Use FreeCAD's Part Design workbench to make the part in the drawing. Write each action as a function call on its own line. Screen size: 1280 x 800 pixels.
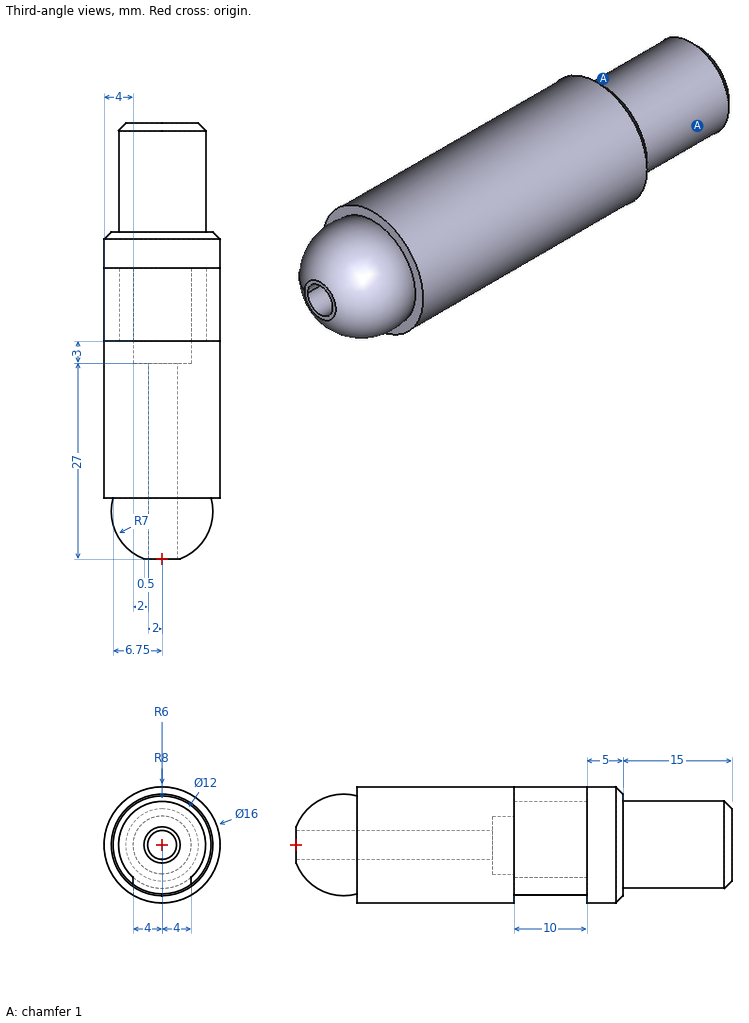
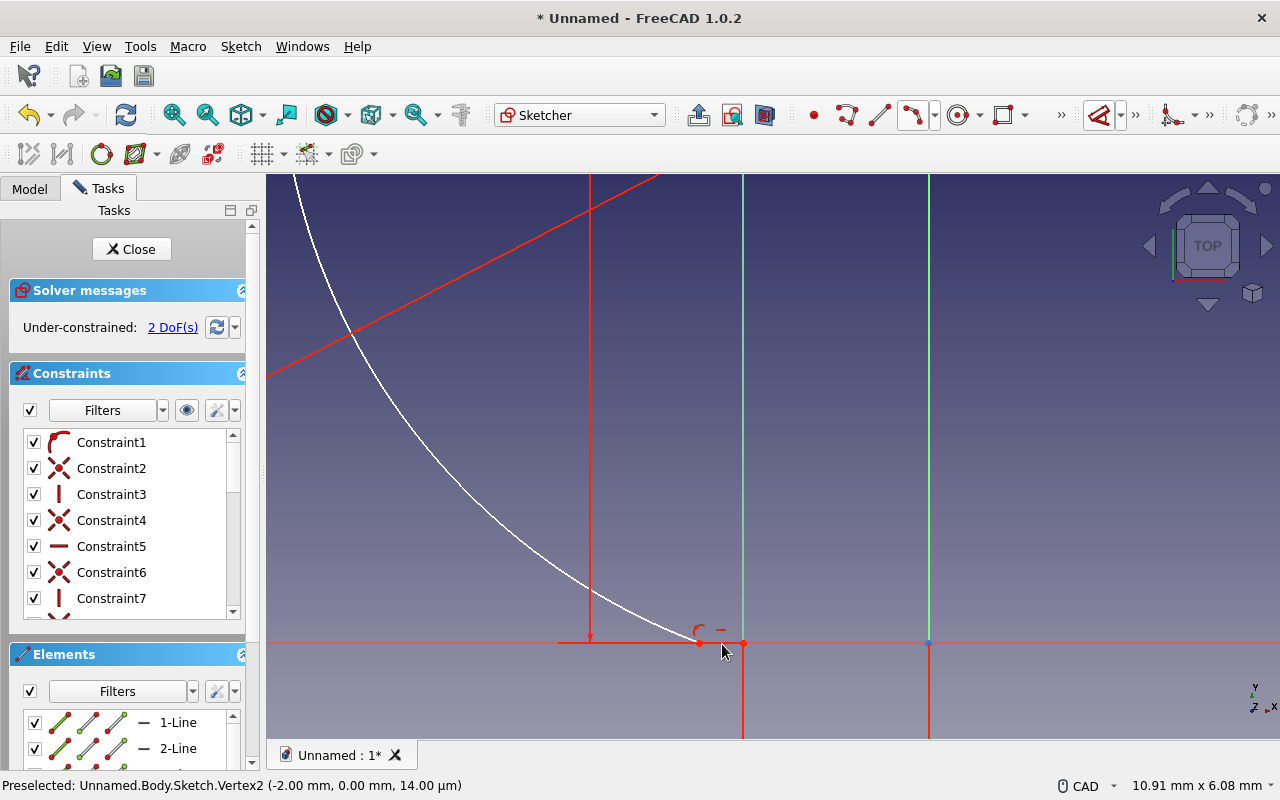
click(722, 643)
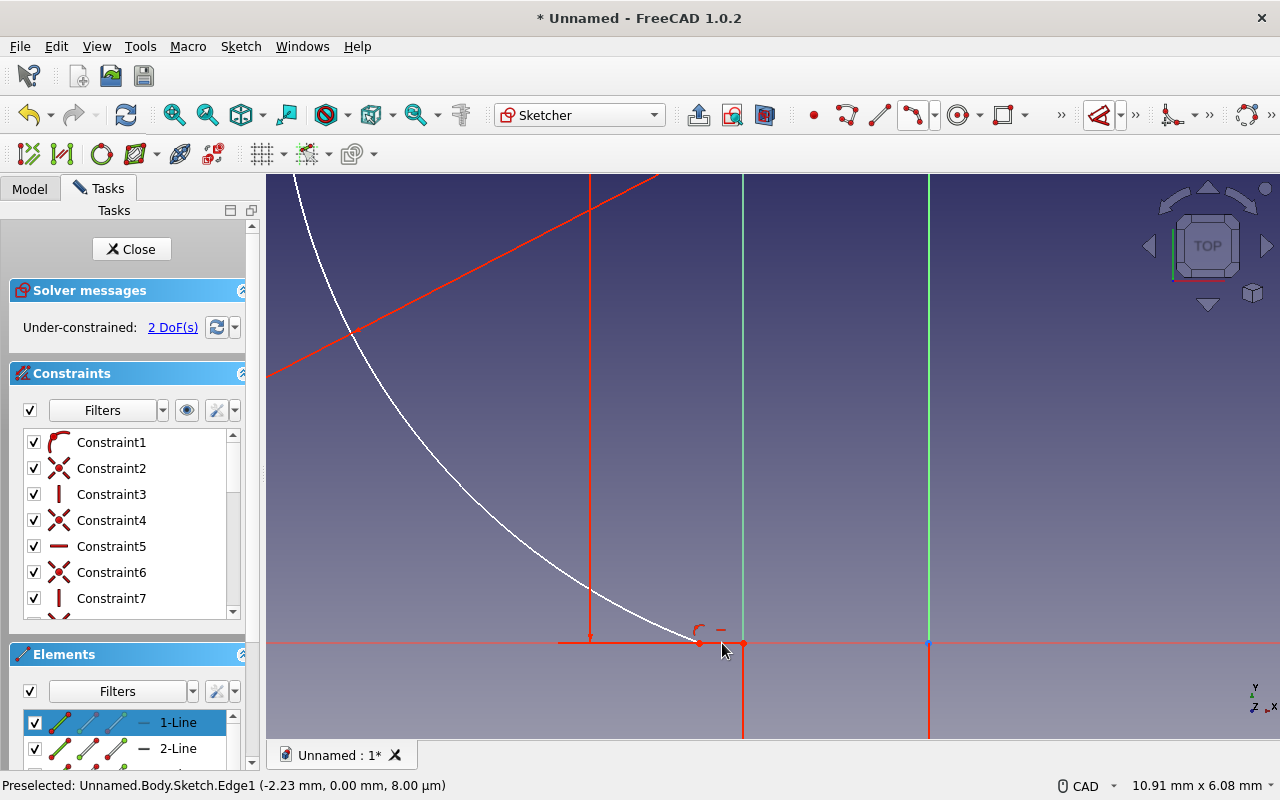
click(1120, 116)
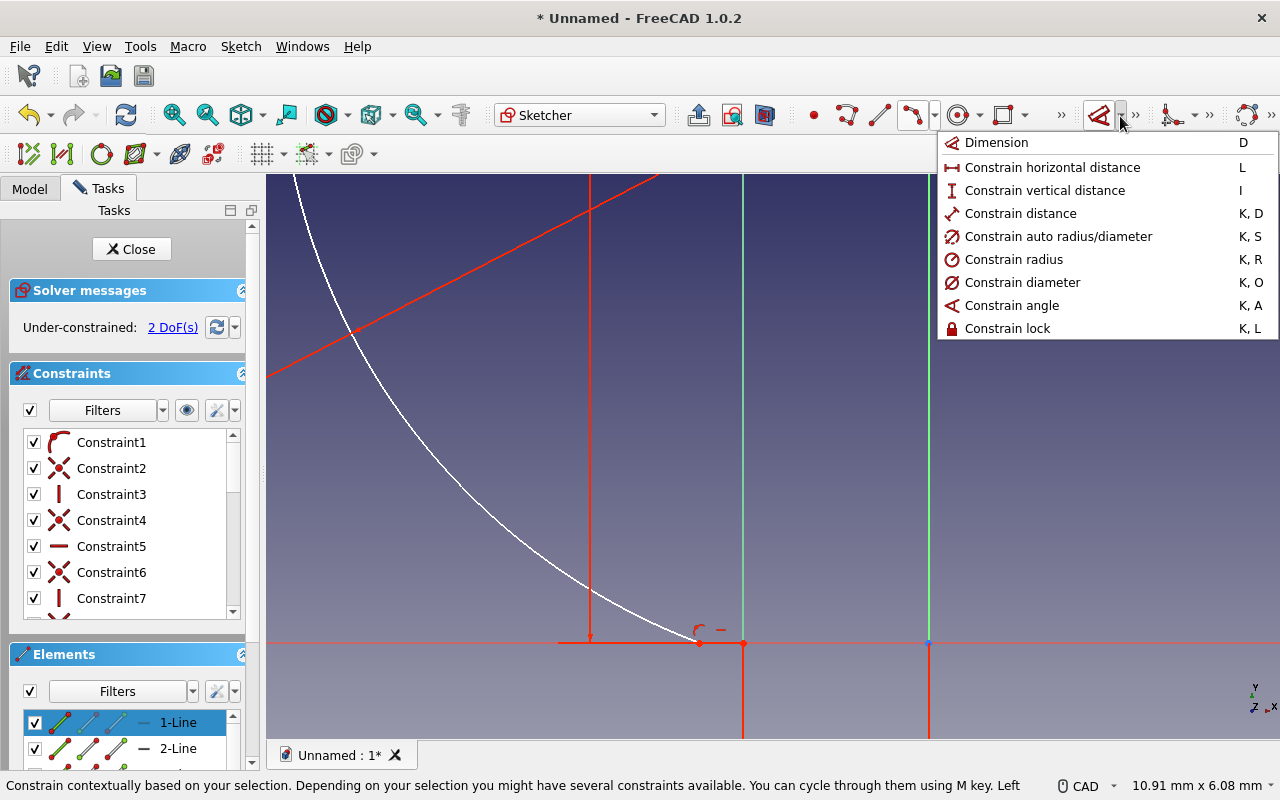
click(1108, 168)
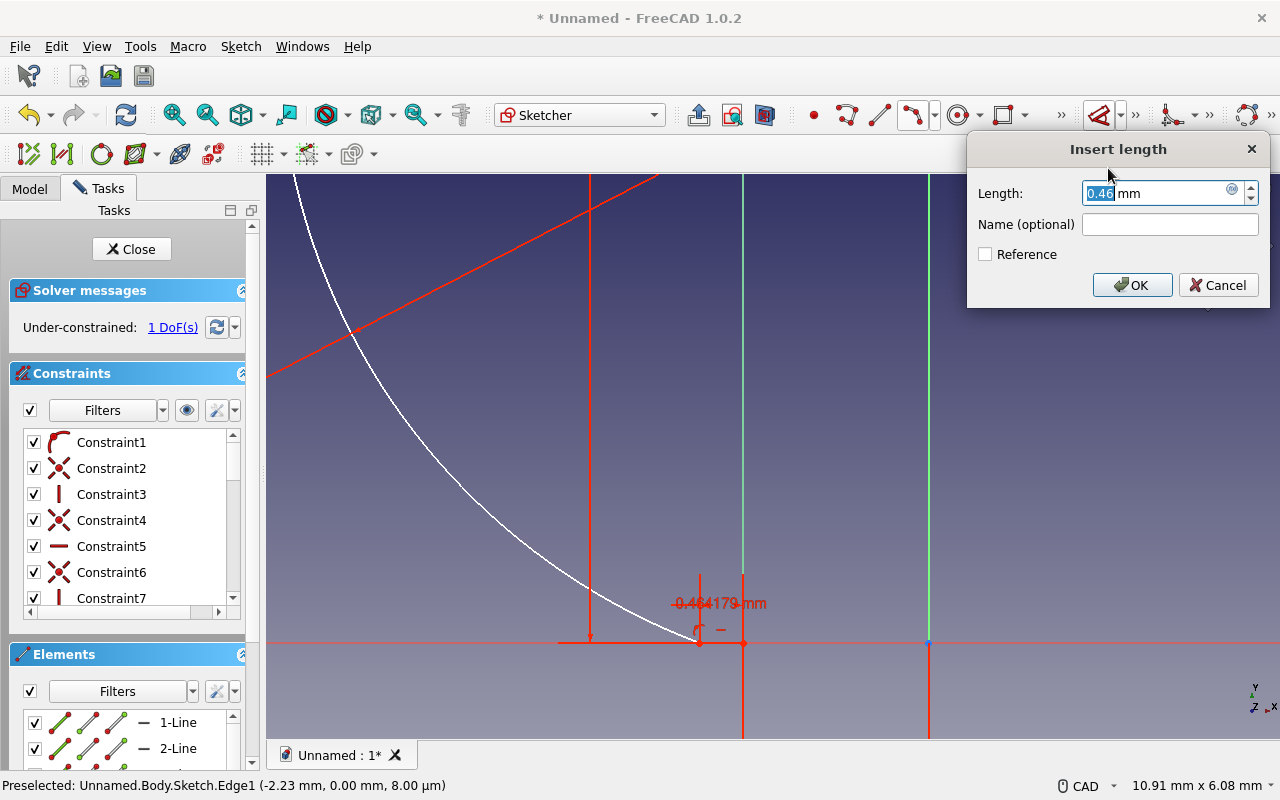
text(0.5)
key(Return)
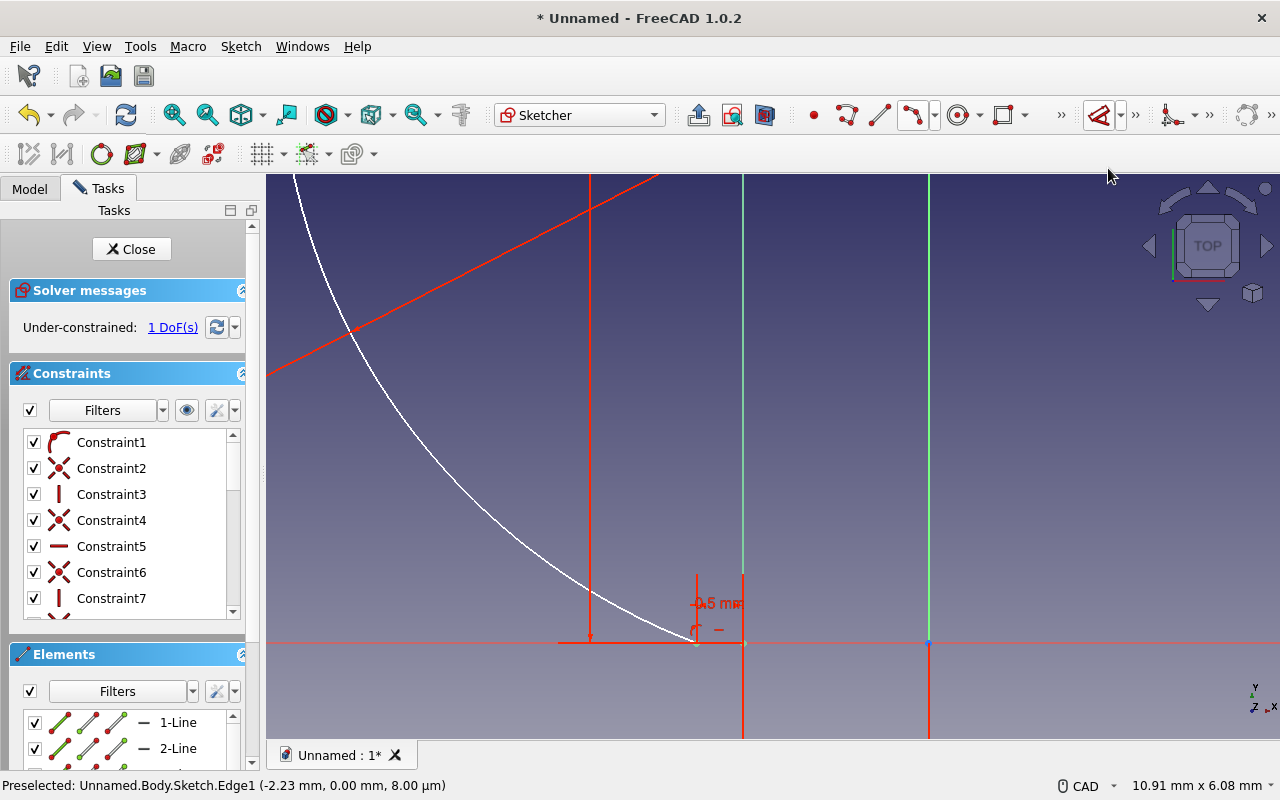
scroll(728, 645, down, 10)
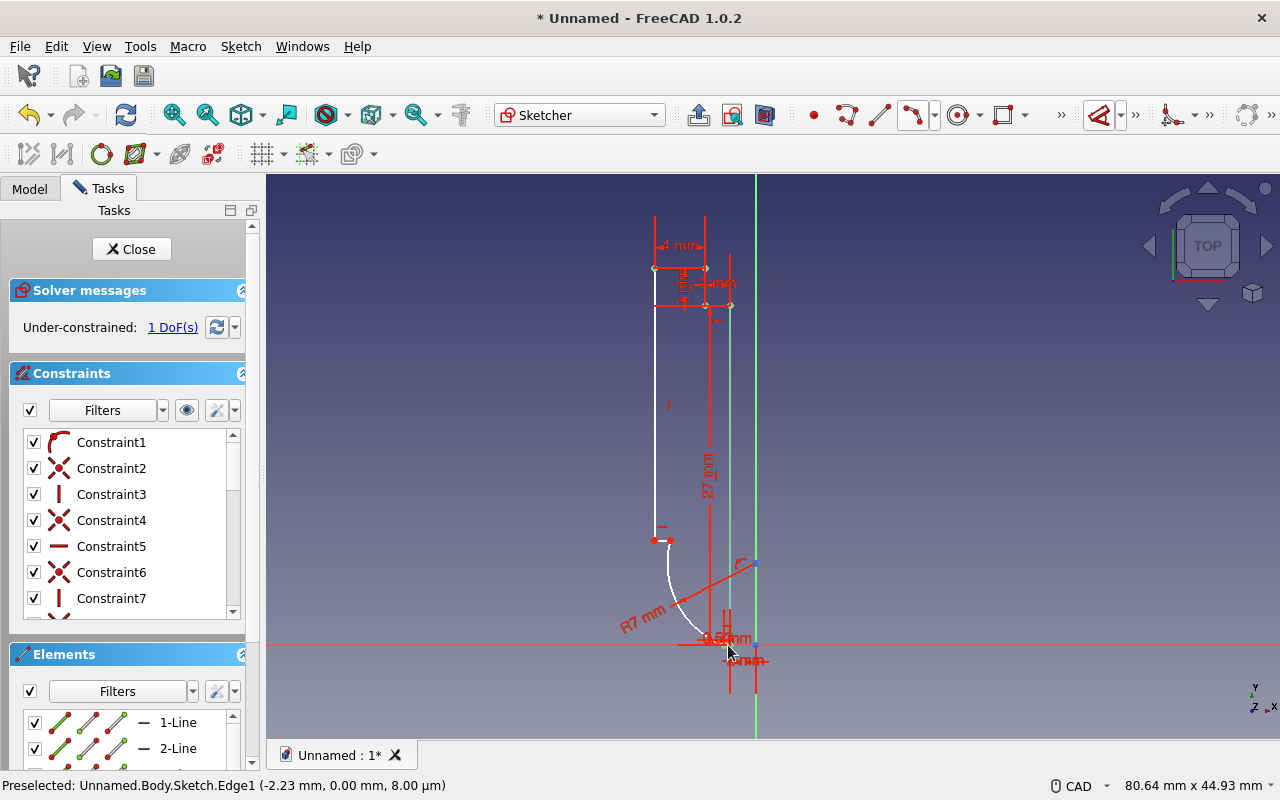
click(670, 541)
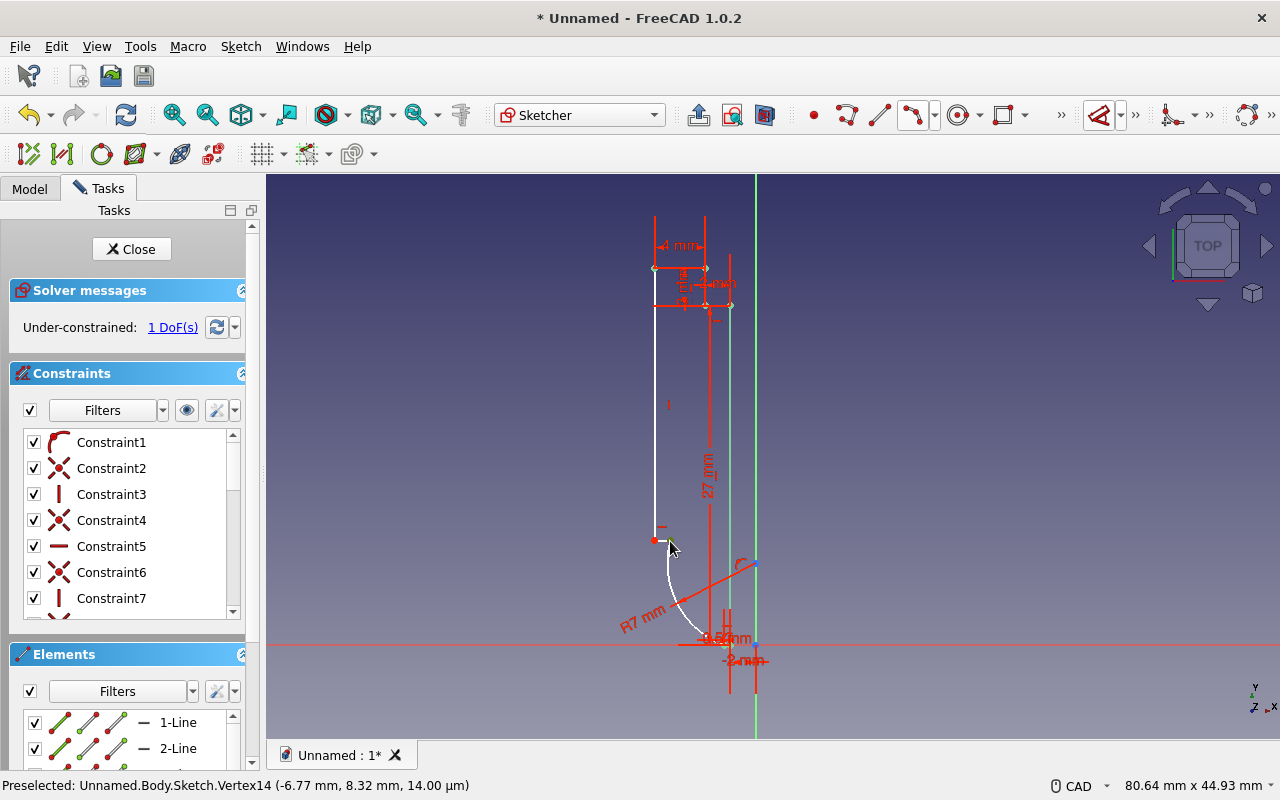
key(l)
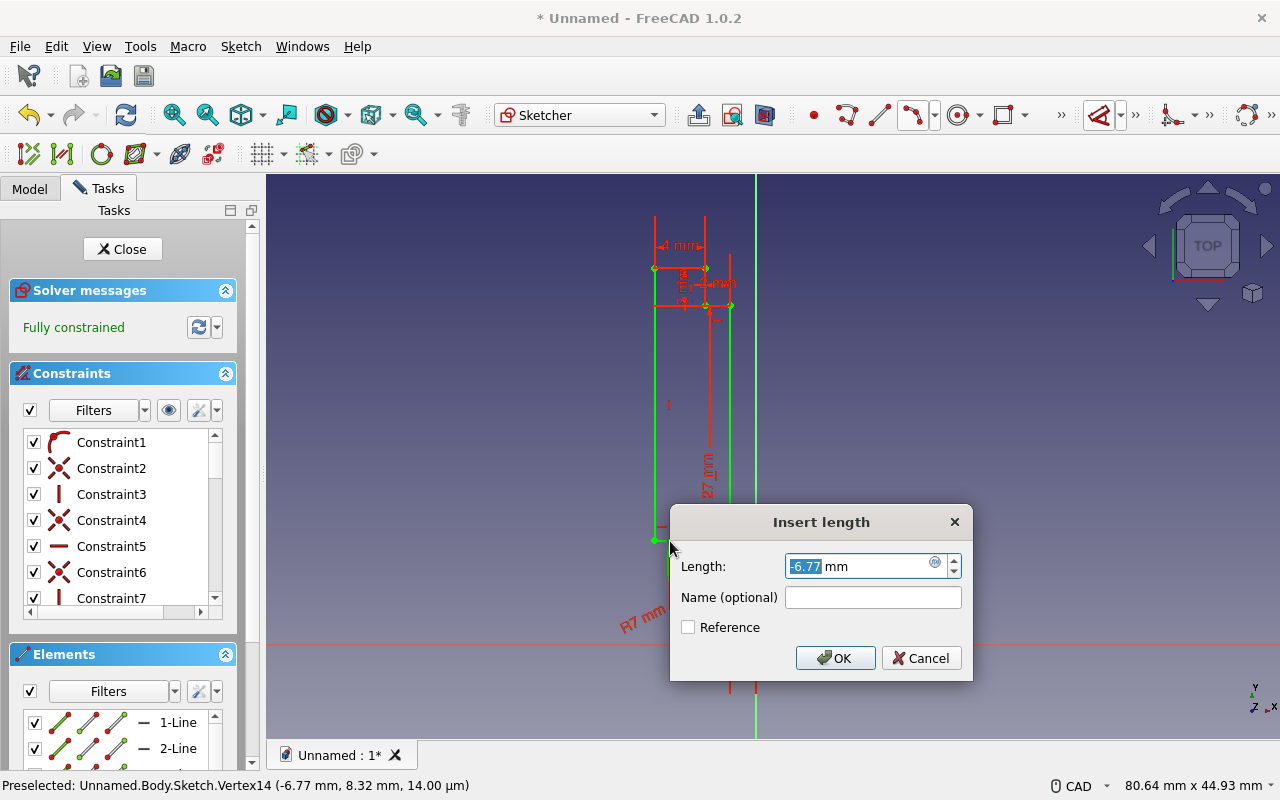
text(-6.75)
key(Return)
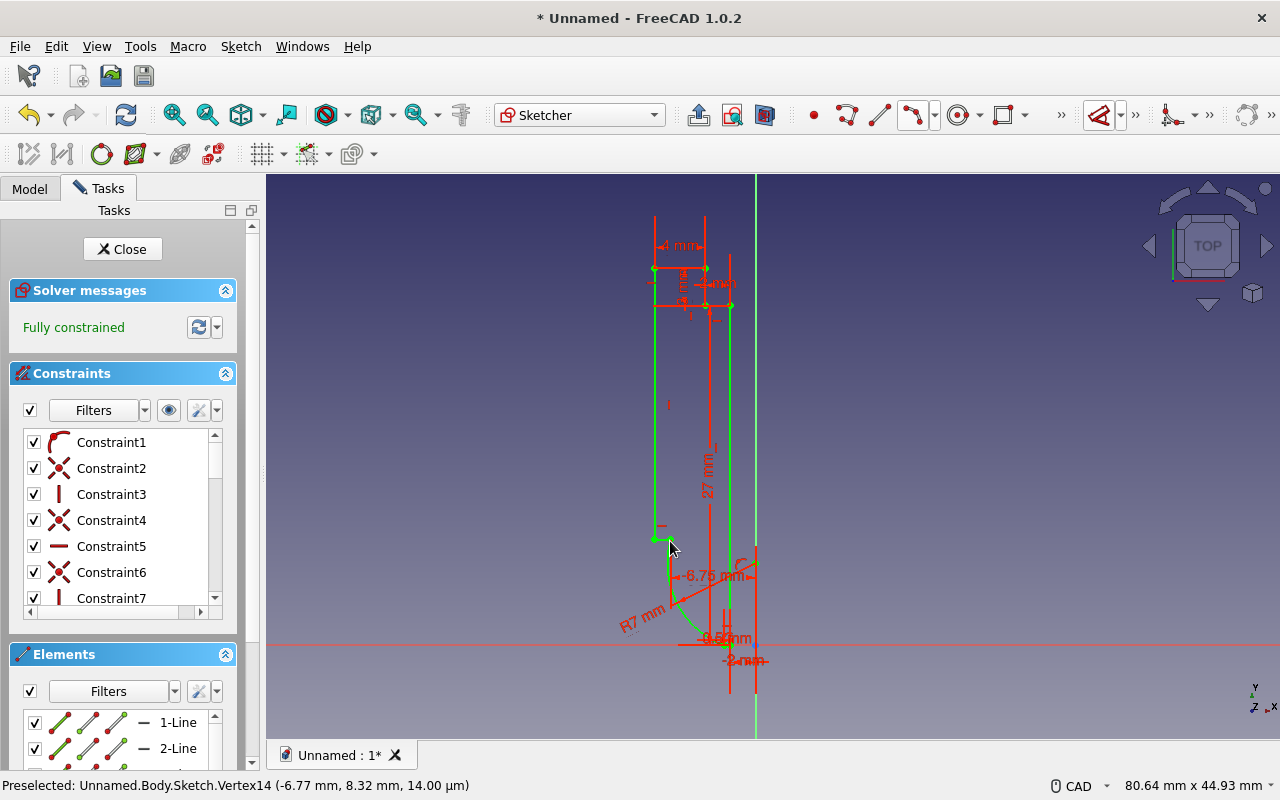
click(123, 249)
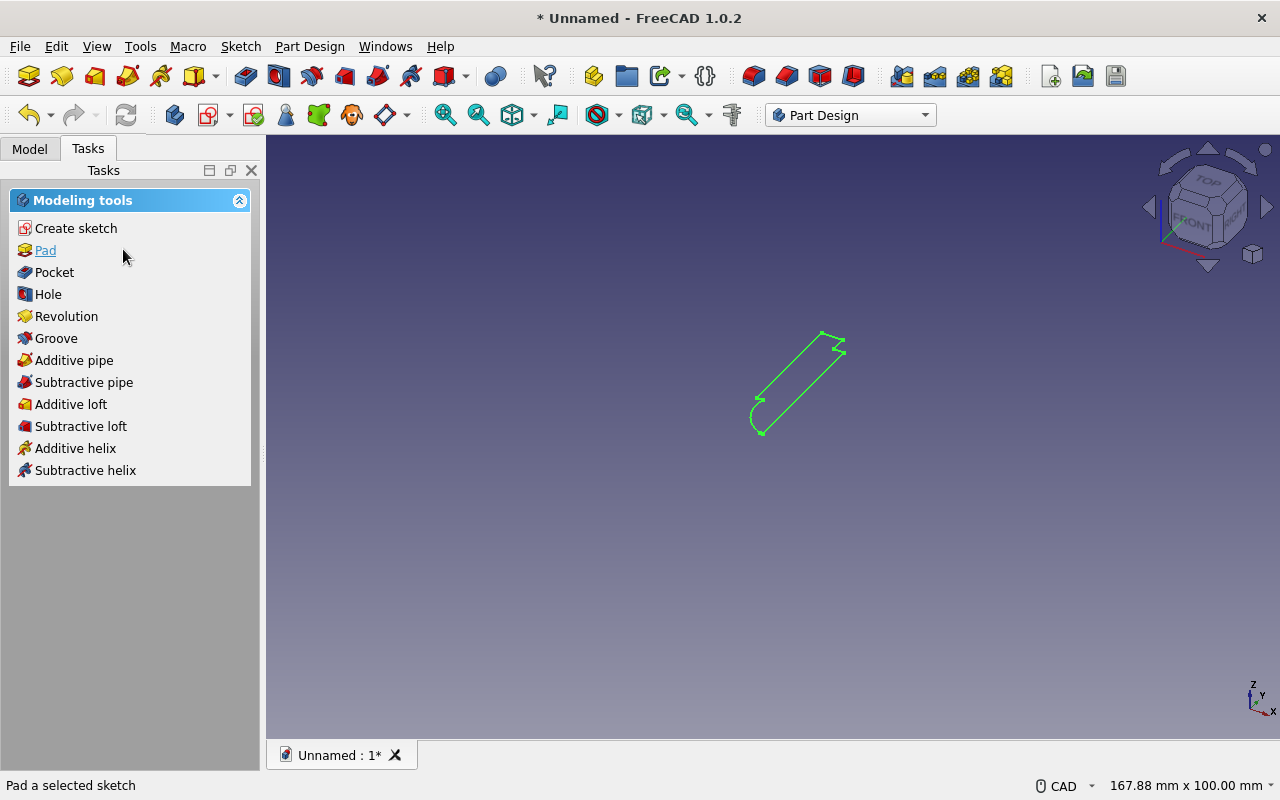
click(62, 76)